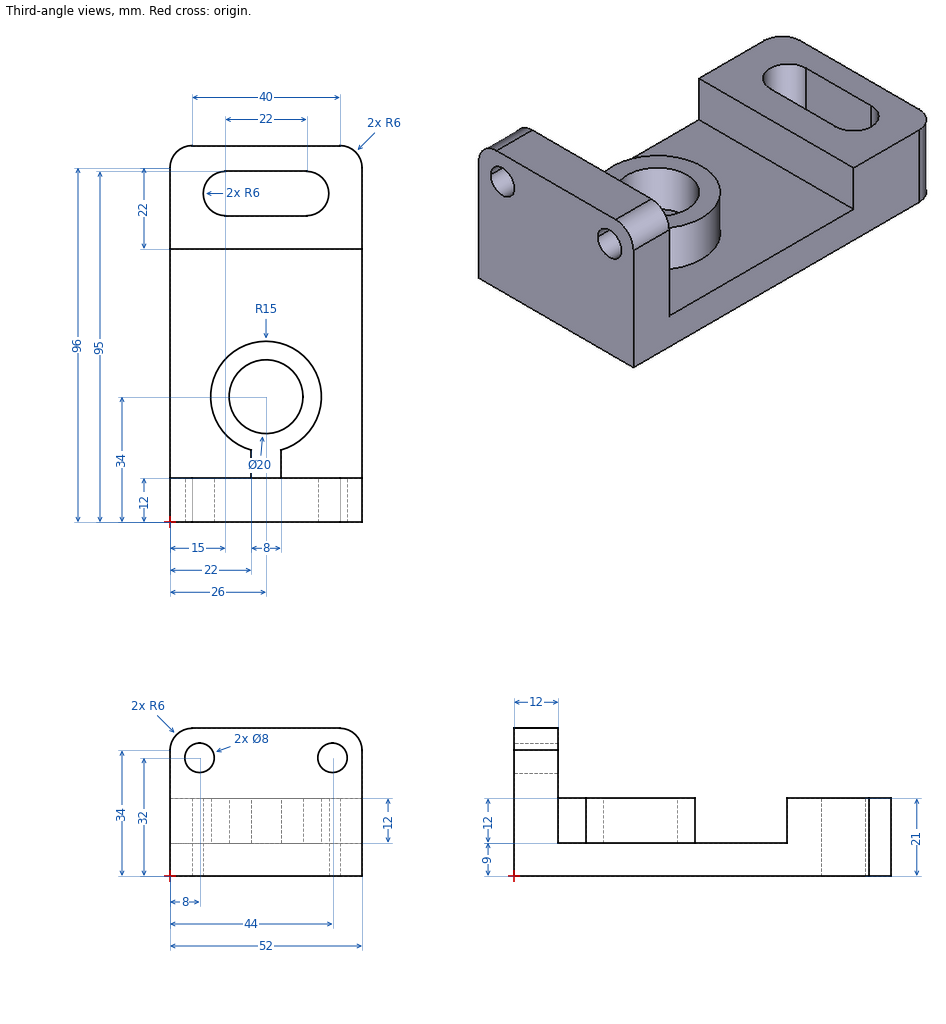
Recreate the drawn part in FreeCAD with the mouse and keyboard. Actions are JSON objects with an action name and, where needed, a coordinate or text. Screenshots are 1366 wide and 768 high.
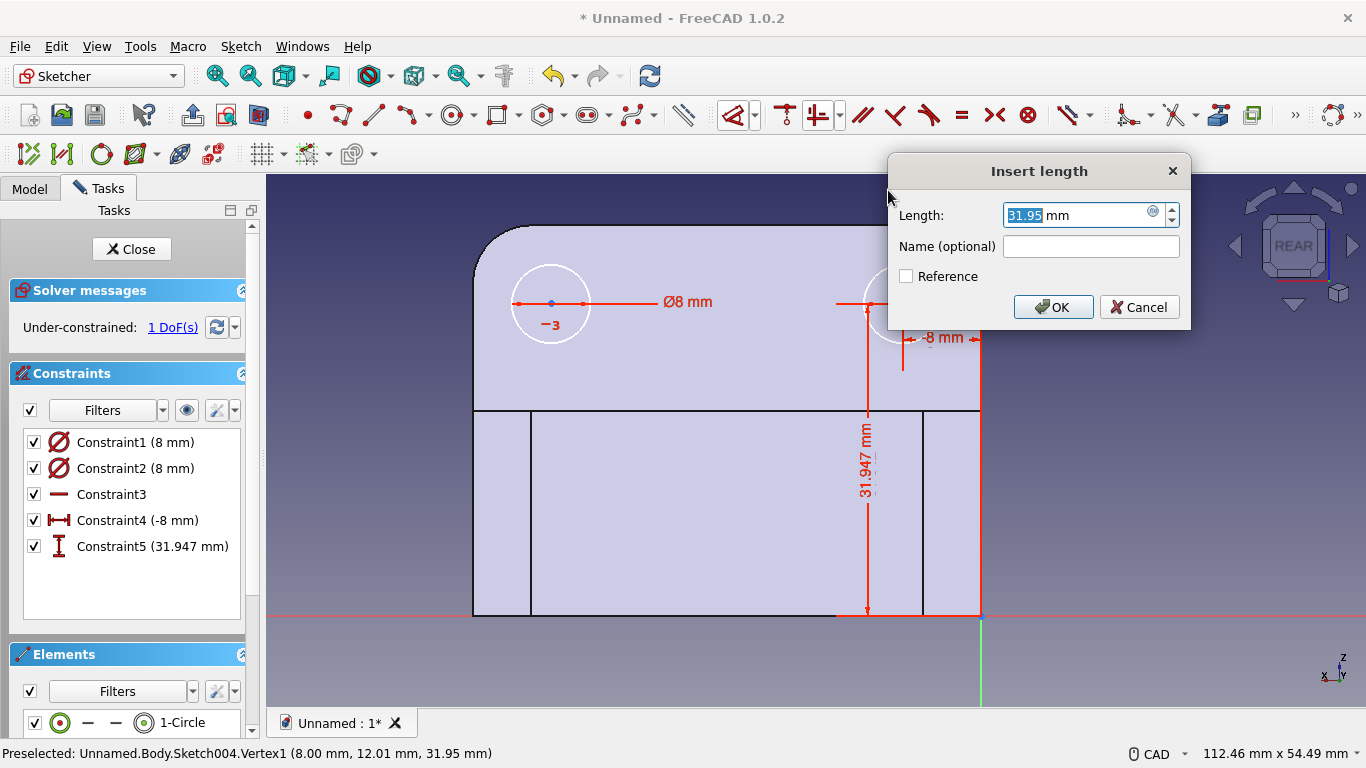
{"action": "type", "text": "32"}
{"action": "key", "text": "Return"}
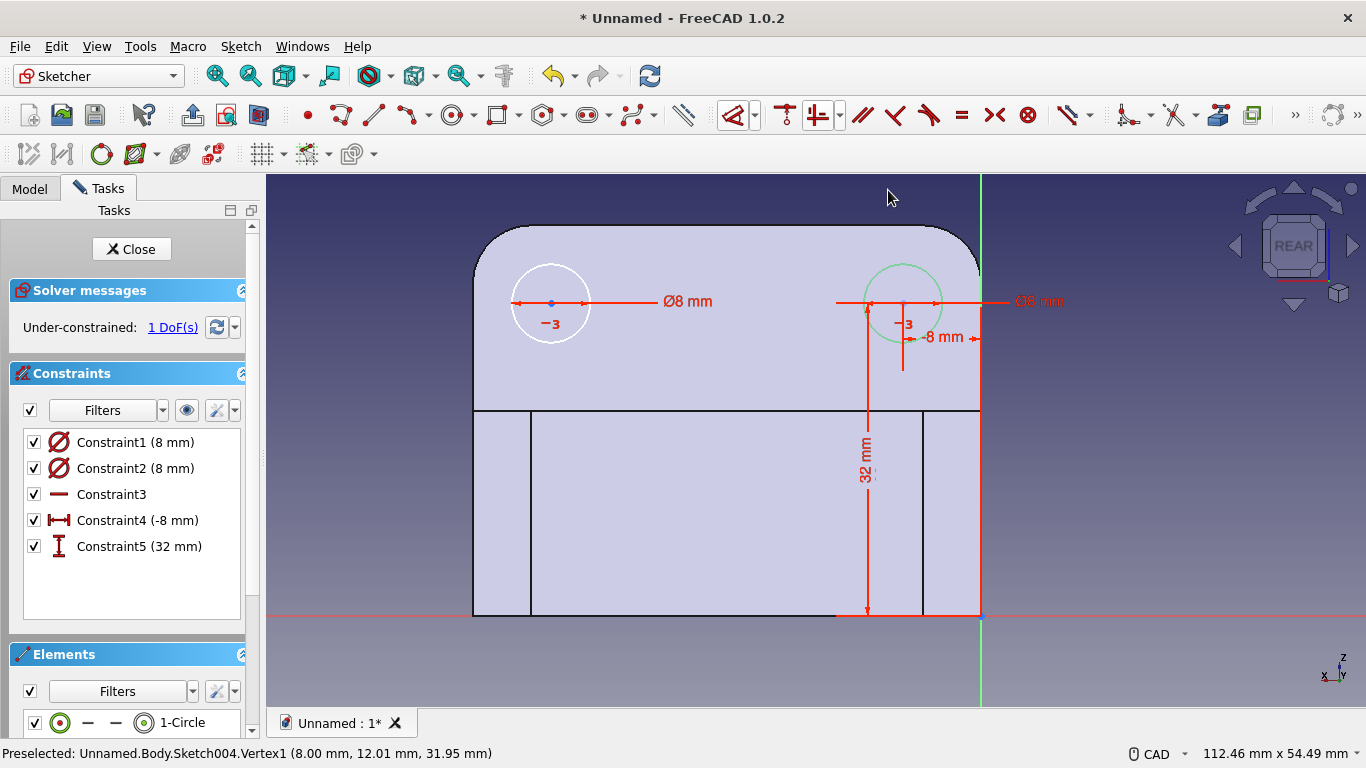
{"action": "left_click", "coordinate": [551, 303]}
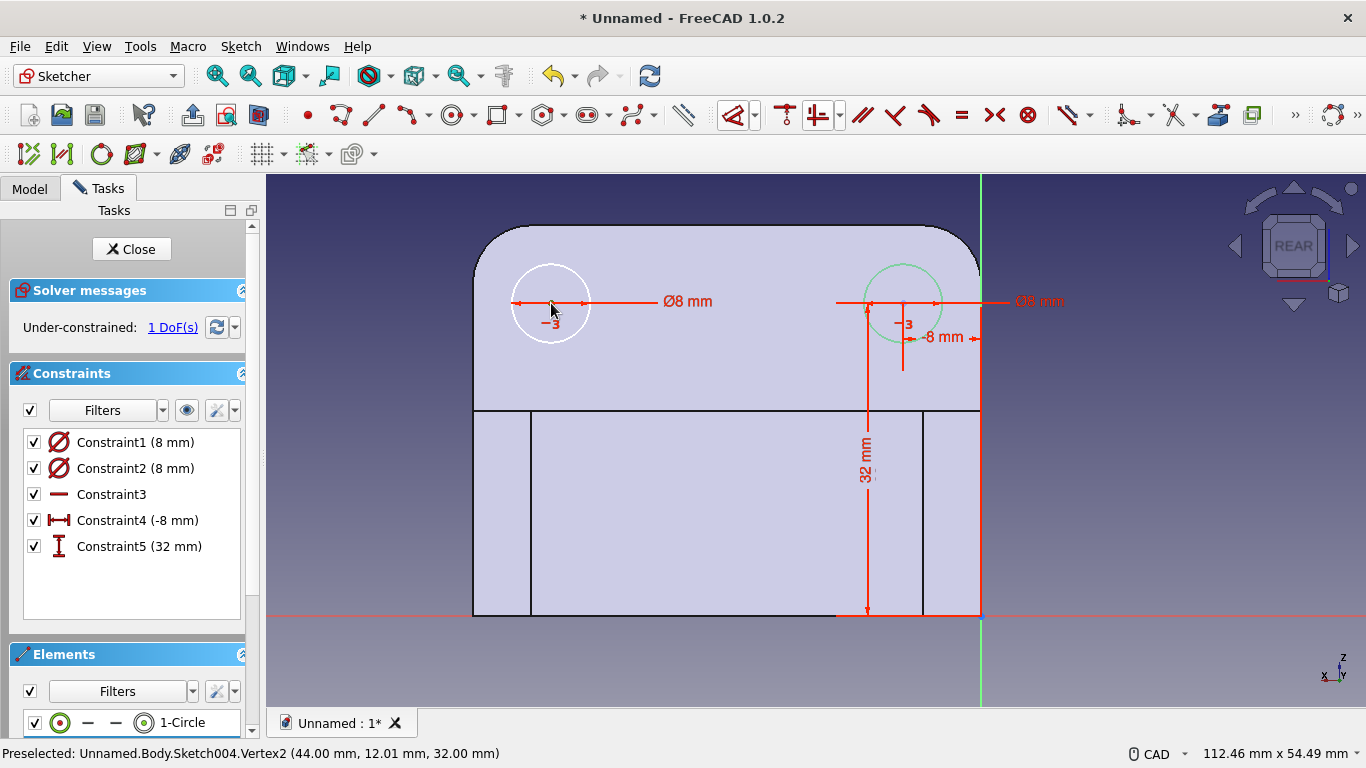
{"action": "key", "text": "l"}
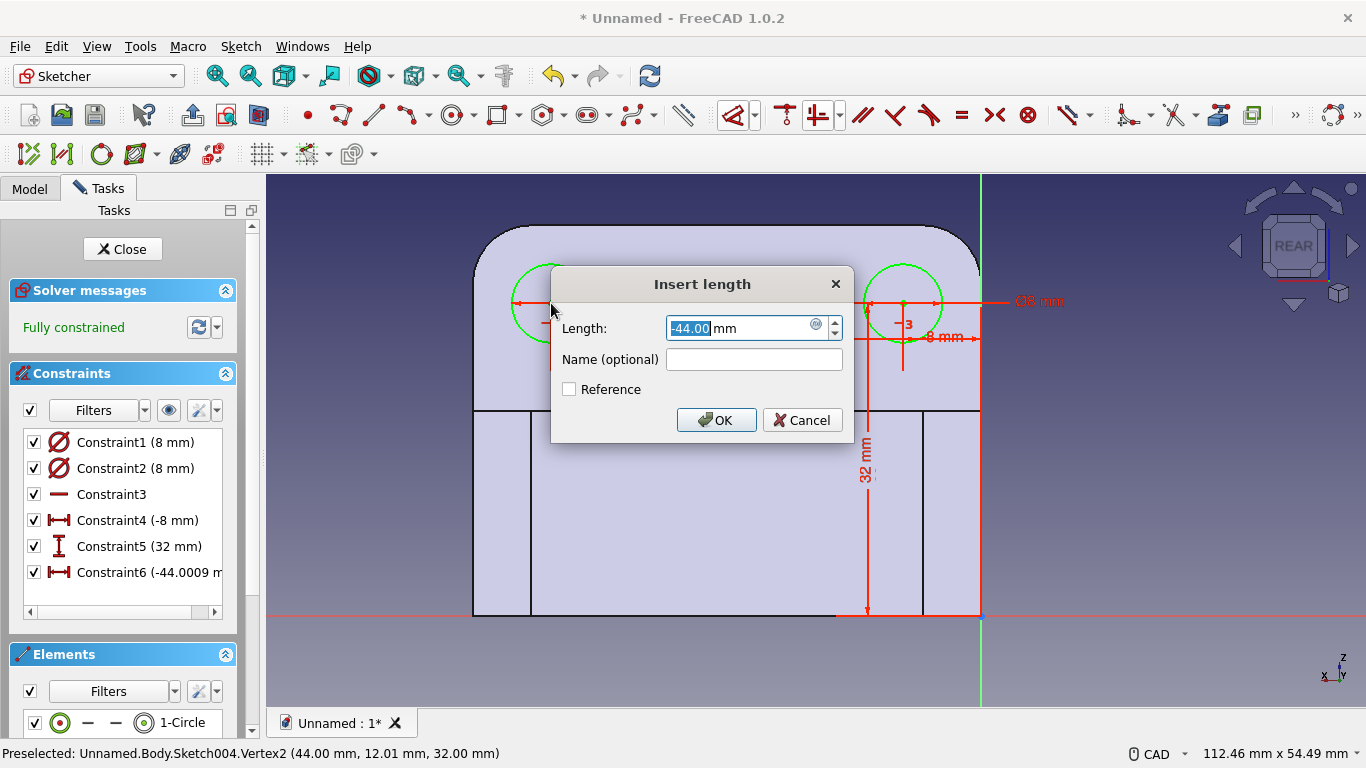
{"action": "type", "text": "-44"}
{"action": "key", "text": "Return"}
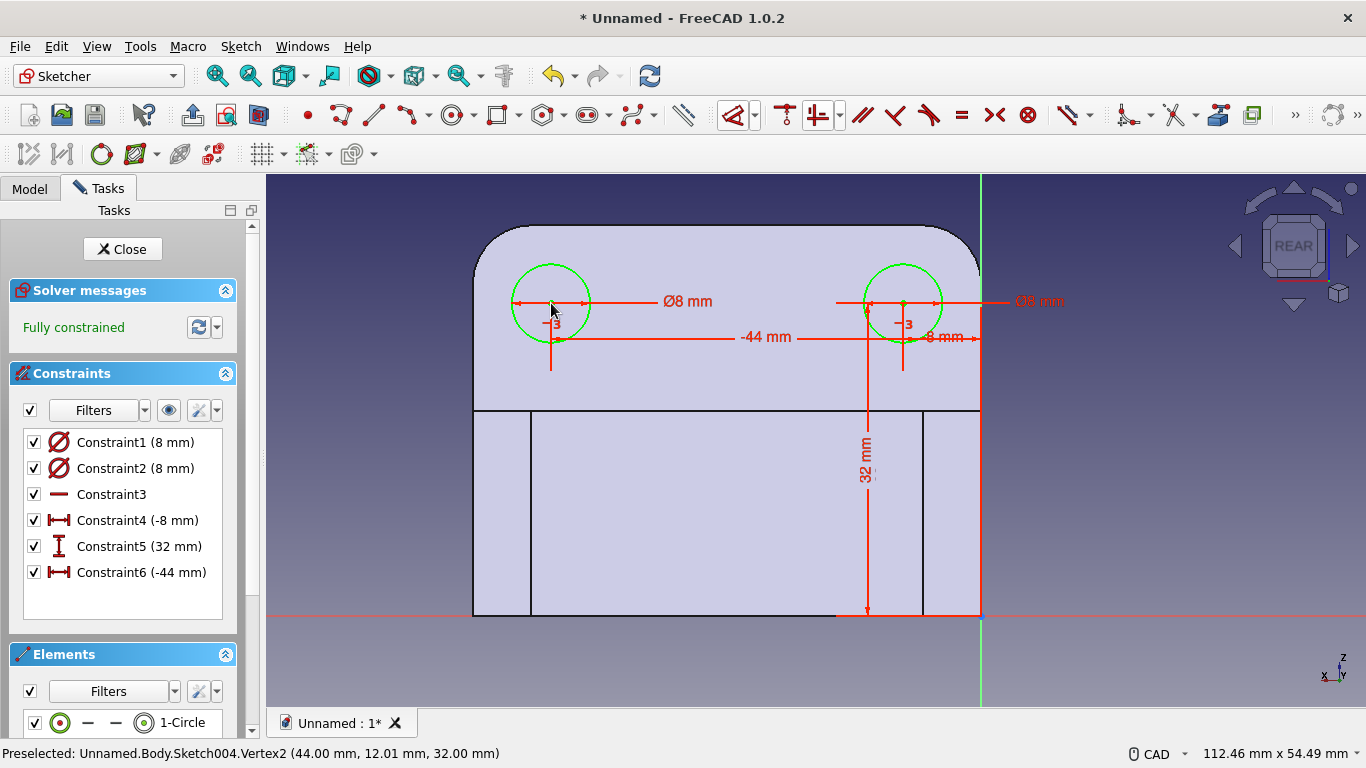
{"action": "left_click", "coordinate": [123, 249]}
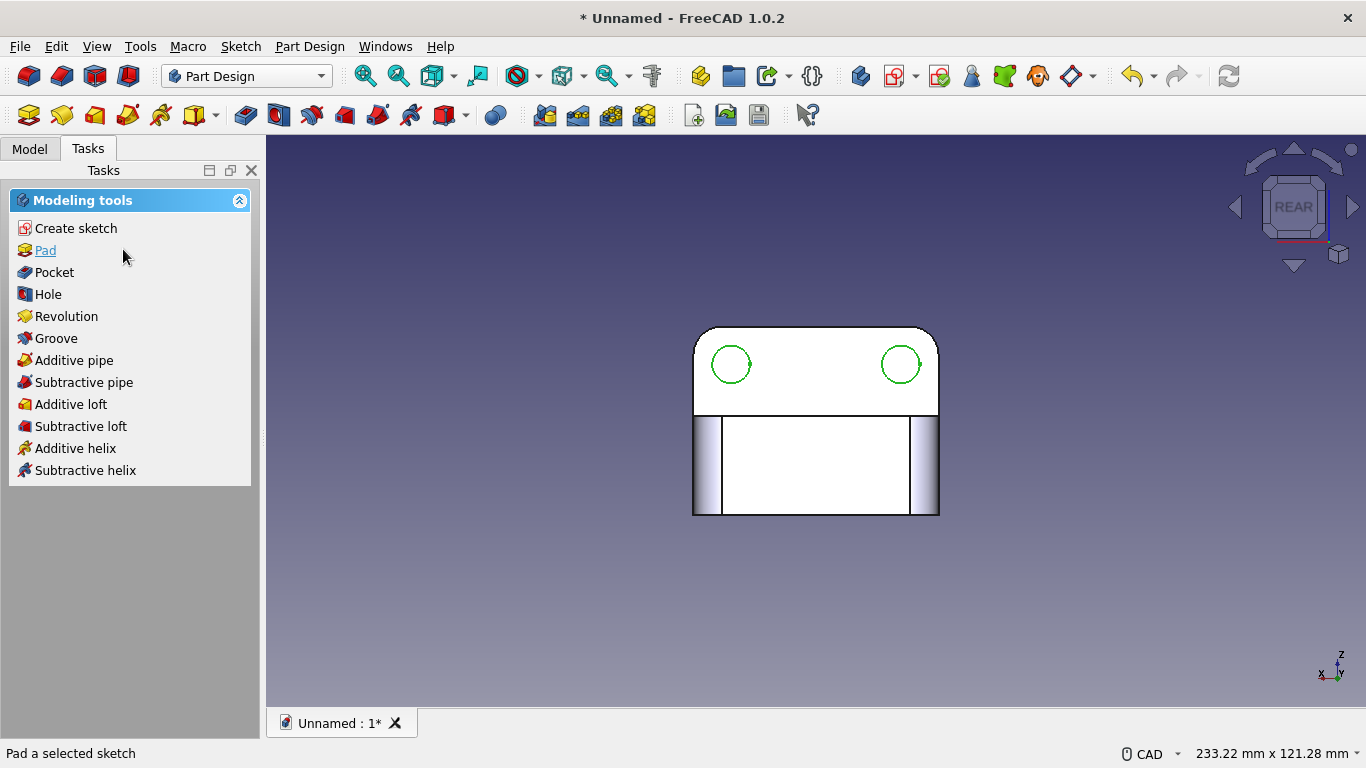
{"action": "left_click", "coordinate": [246, 116]}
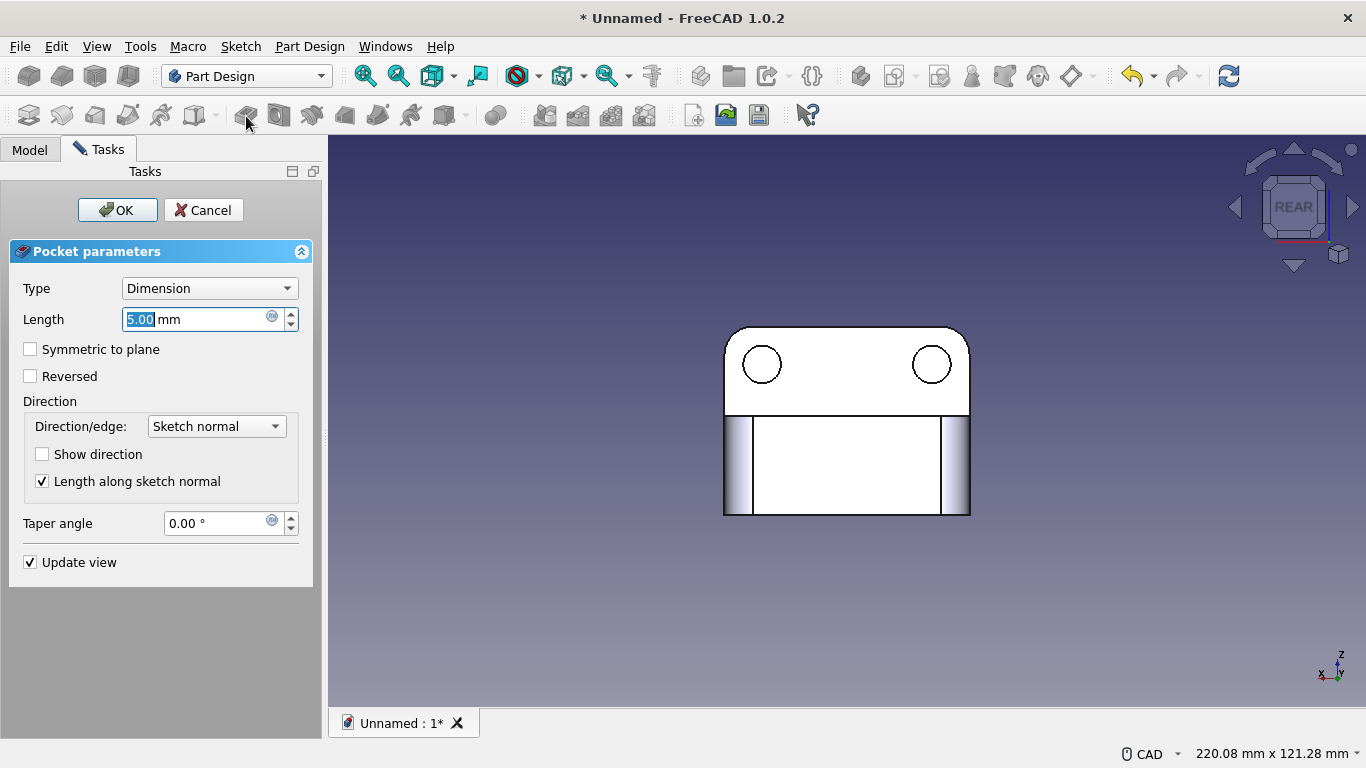
{"action": "type", "text": "12"}
{"action": "key", "text": "Tab"}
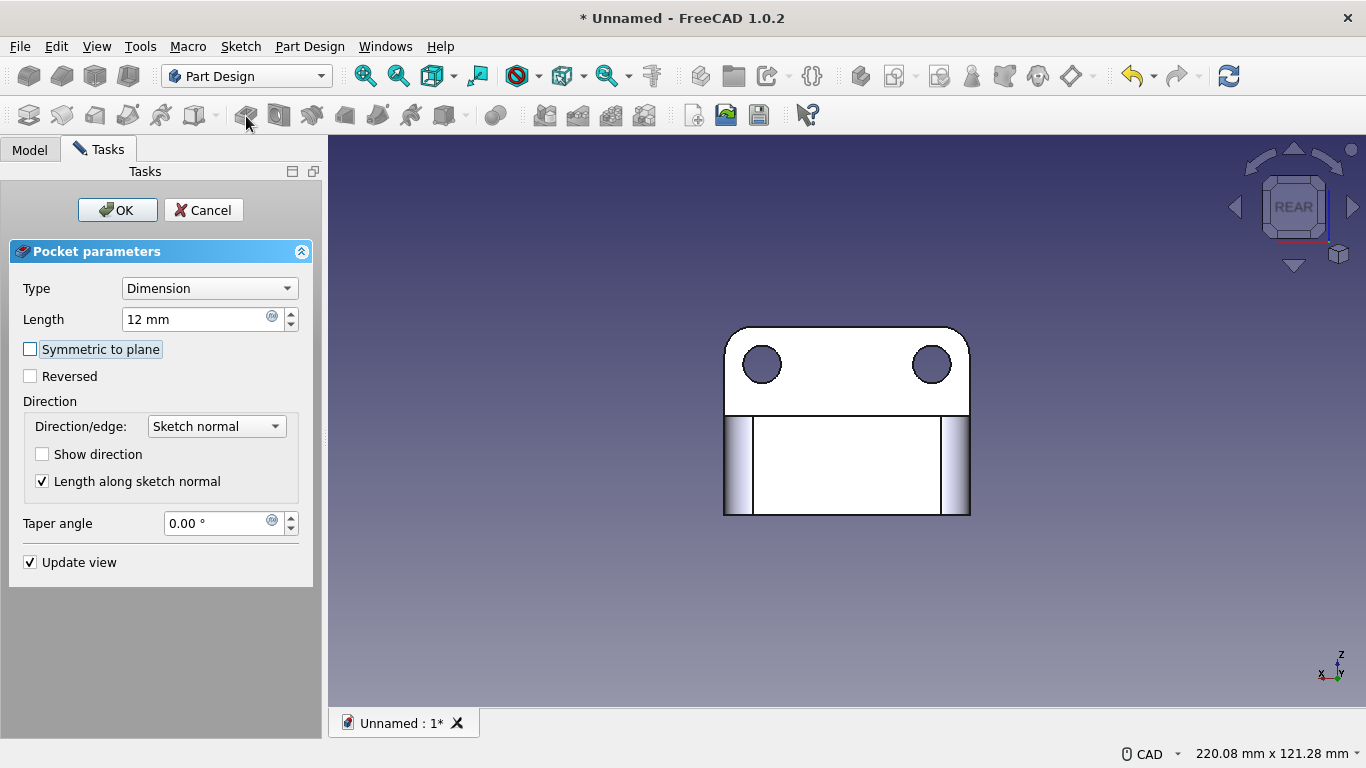
{"action": "left_click", "coordinate": [118, 210]}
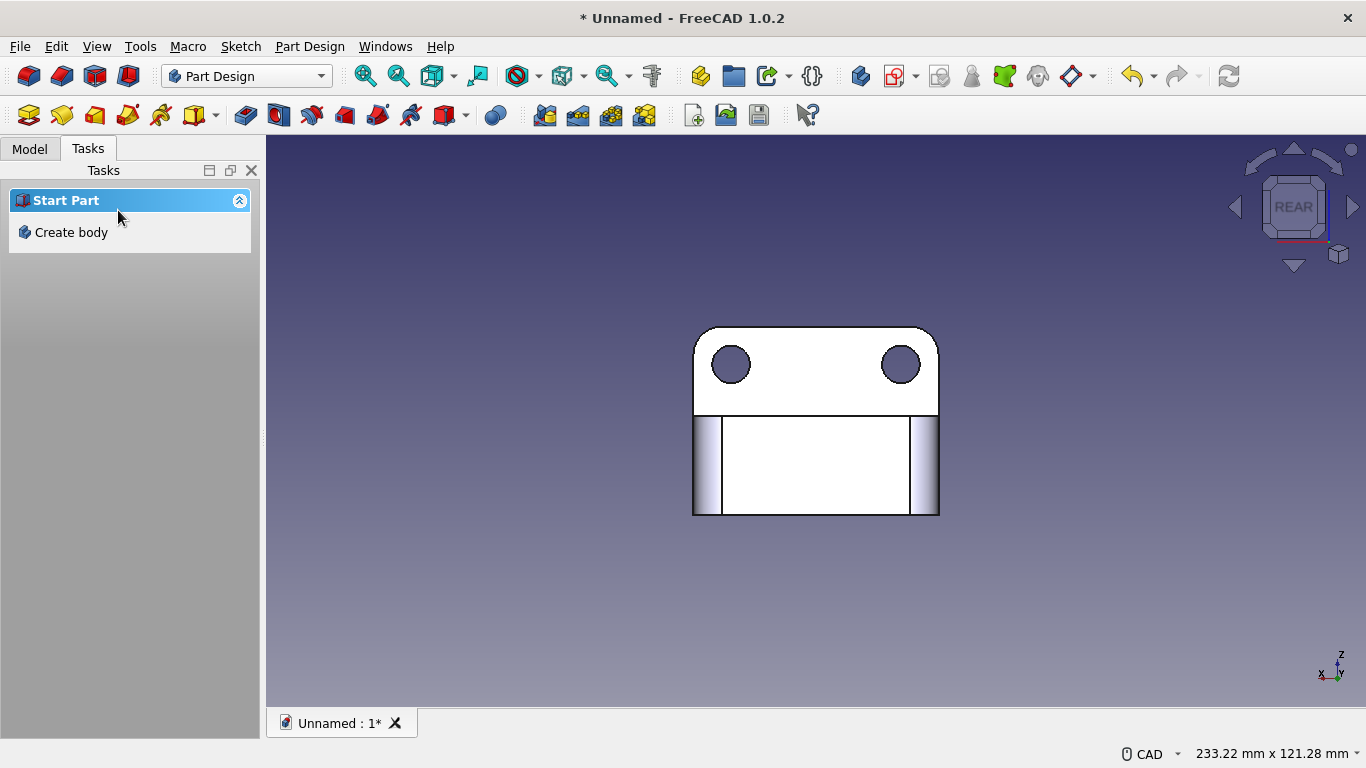
{"action": "left_click", "coordinate": [366, 76]}